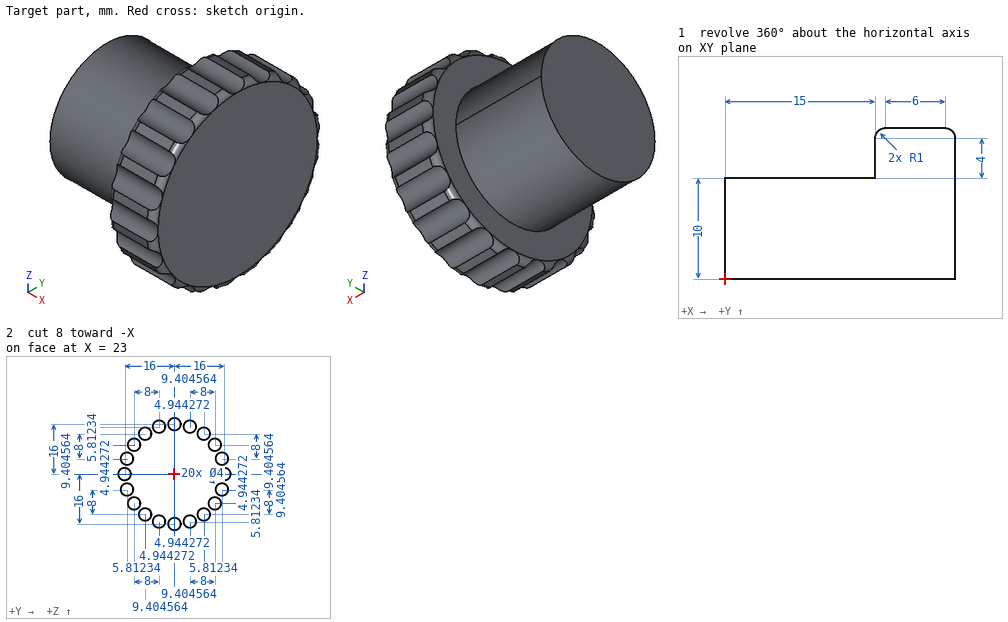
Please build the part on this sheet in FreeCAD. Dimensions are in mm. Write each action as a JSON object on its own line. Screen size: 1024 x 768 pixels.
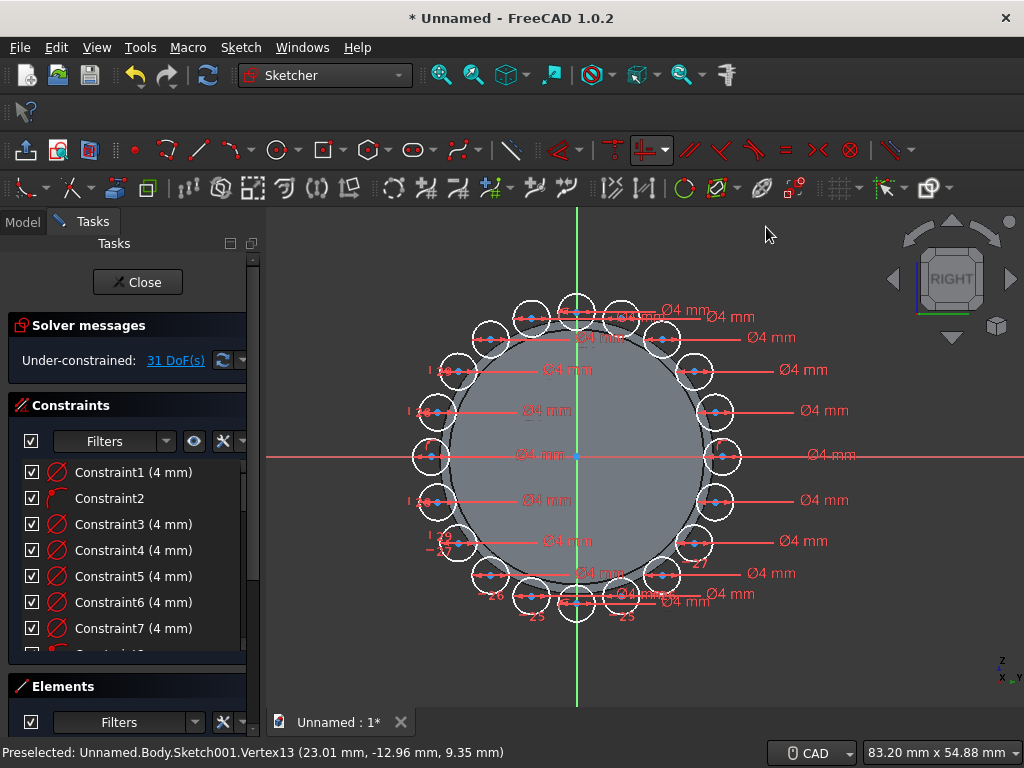
{"action": "left_click", "coordinate": [491, 575]}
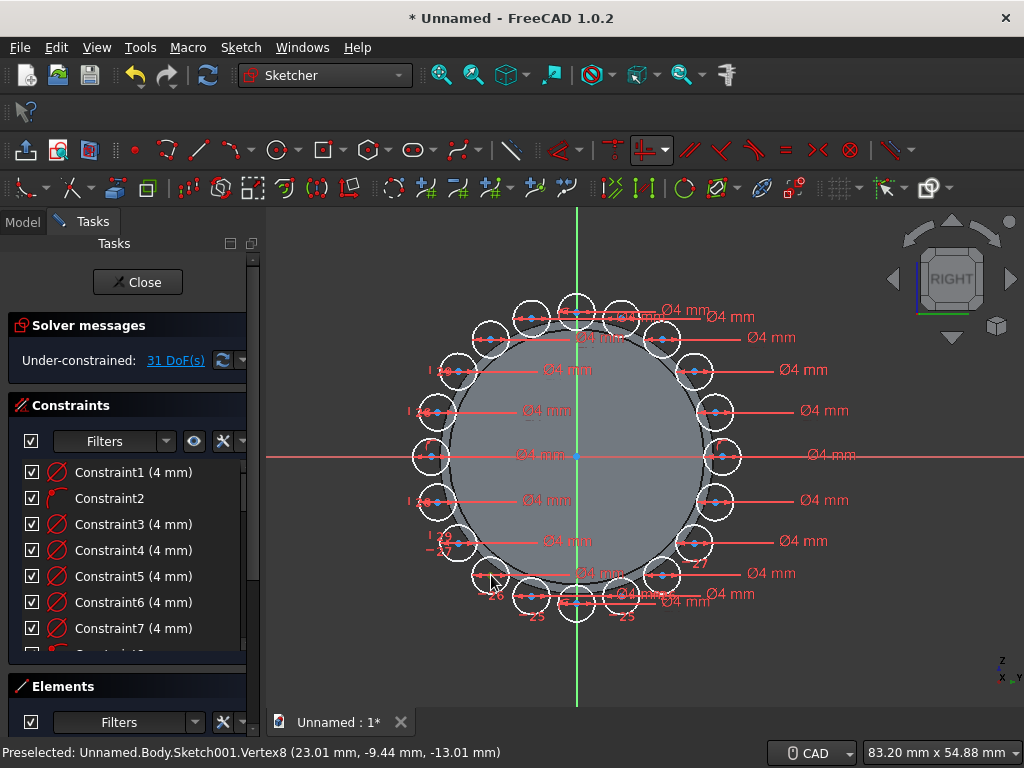
{"action": "left_click", "coordinate": [491, 340]}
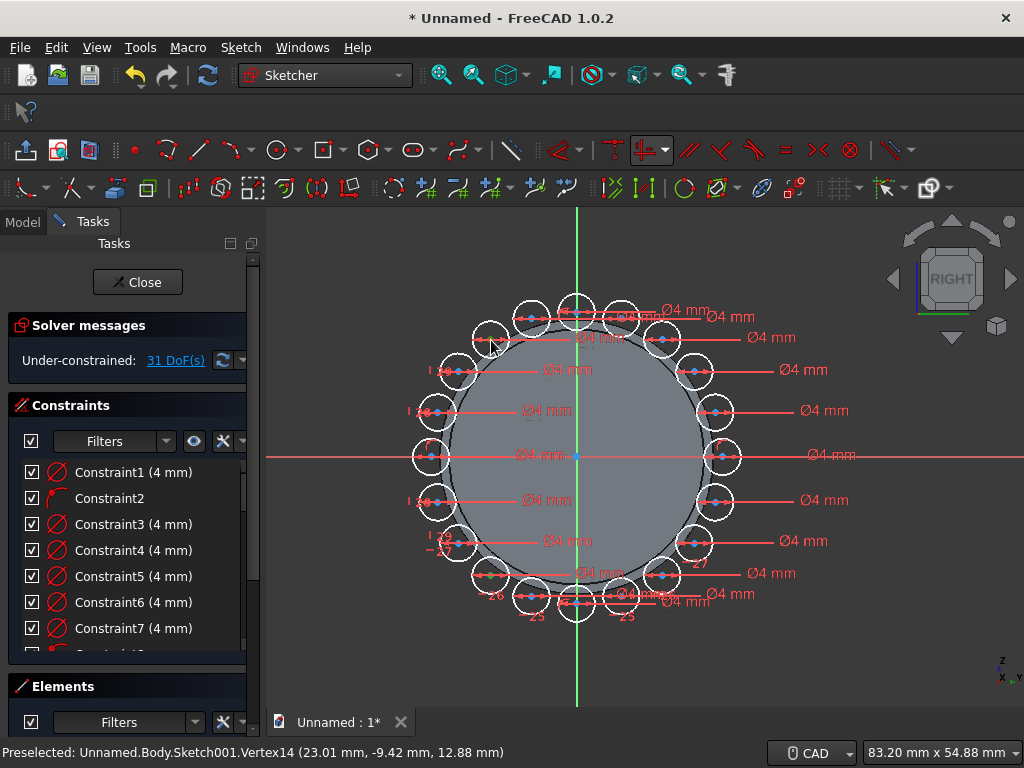
{"action": "left_click", "coordinate": [668, 150]}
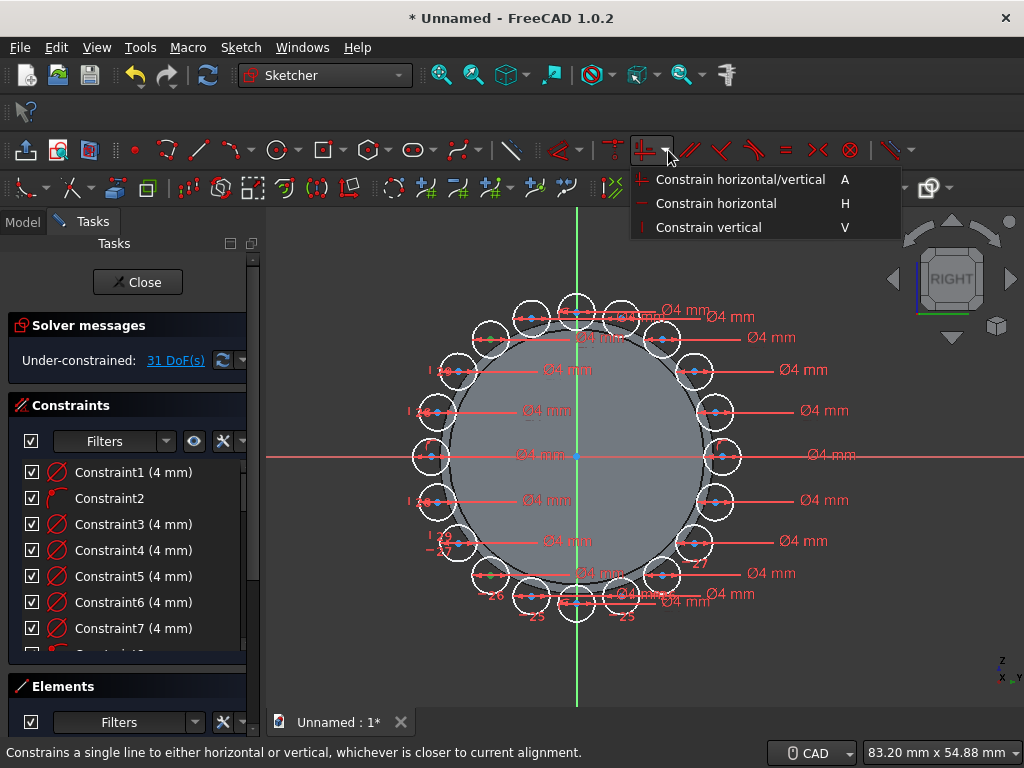
{"action": "left_click", "coordinate": [766, 227]}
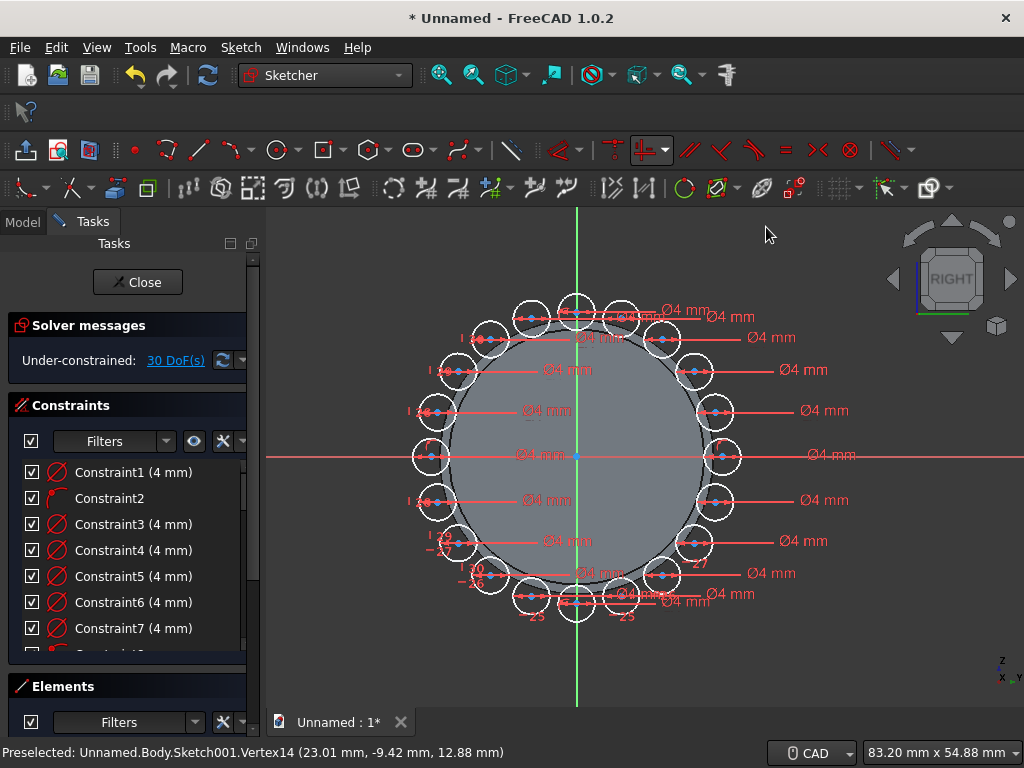
{"action": "left_click", "coordinate": [532, 319]}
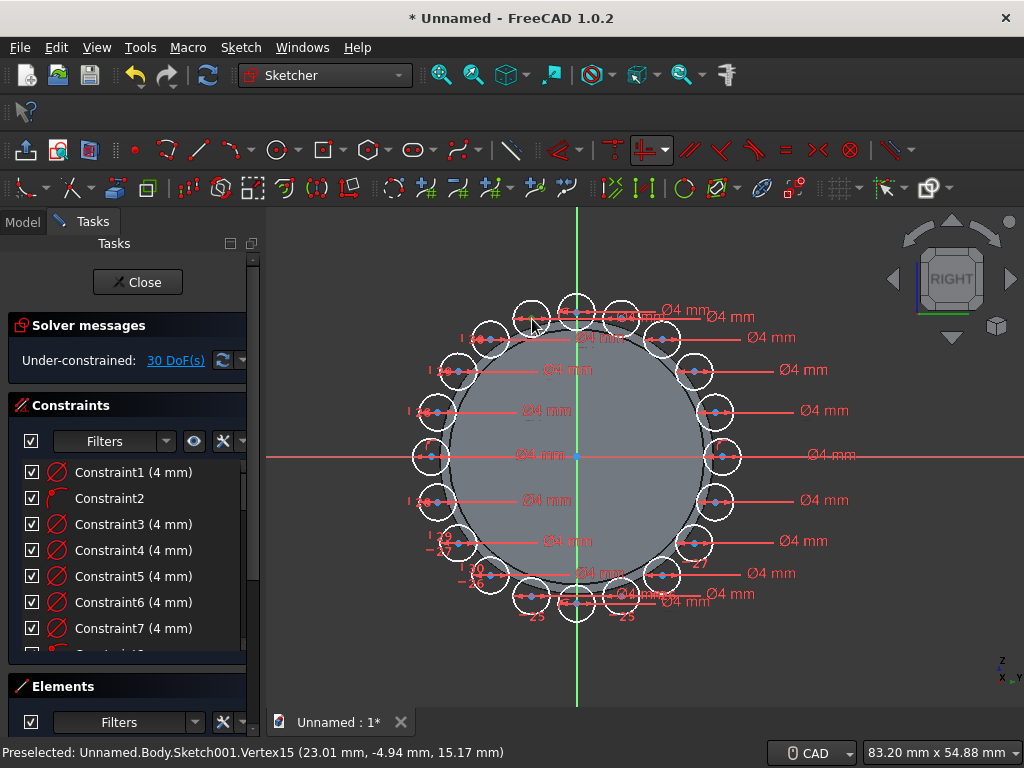
{"action": "left_click", "coordinate": [621, 319]}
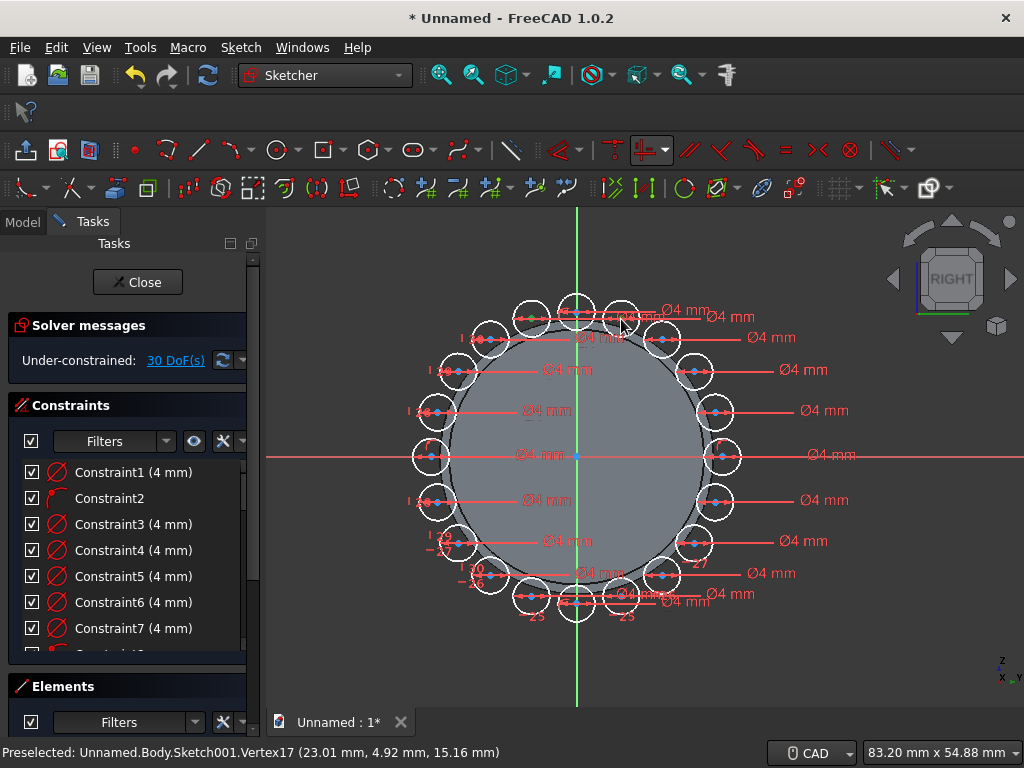
{"action": "left_click", "coordinate": [668, 150]}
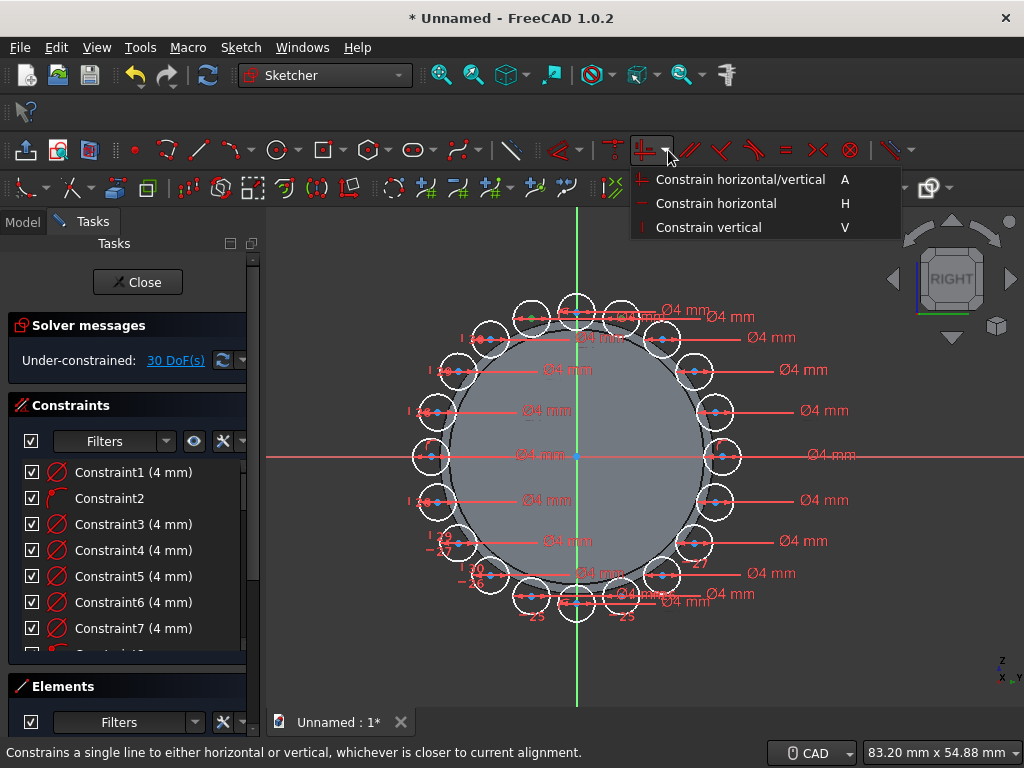
{"action": "left_click", "coordinate": [766, 203]}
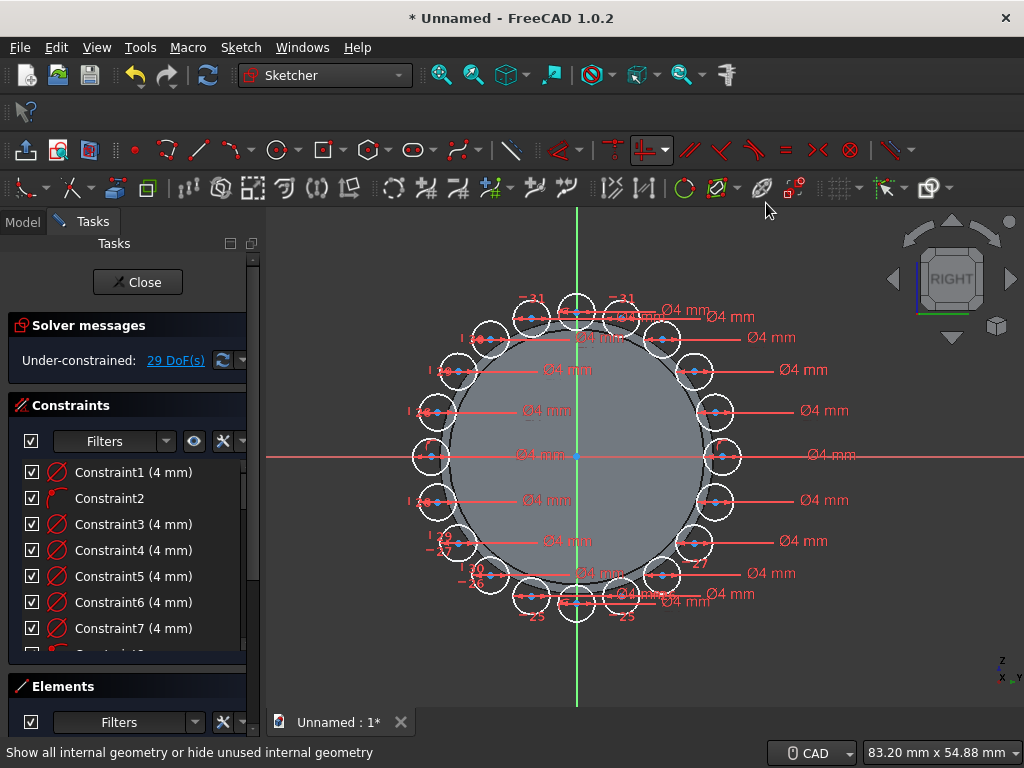
{"action": "left_click", "coordinate": [491, 340]}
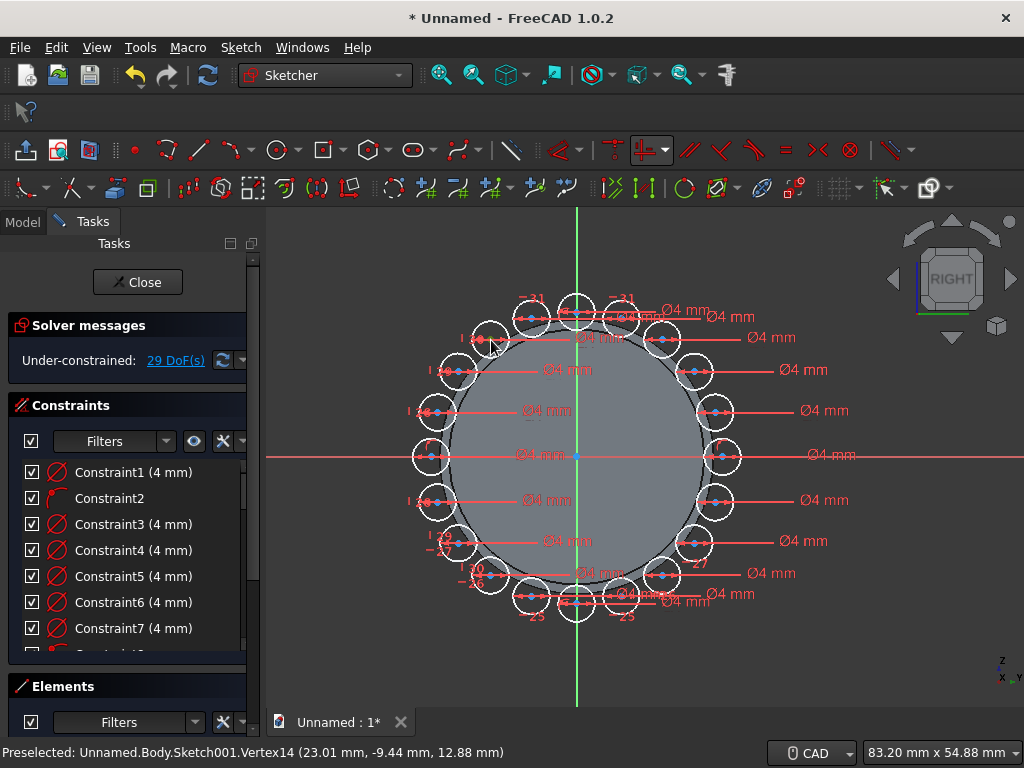
{"action": "left_click", "coordinate": [662, 340]}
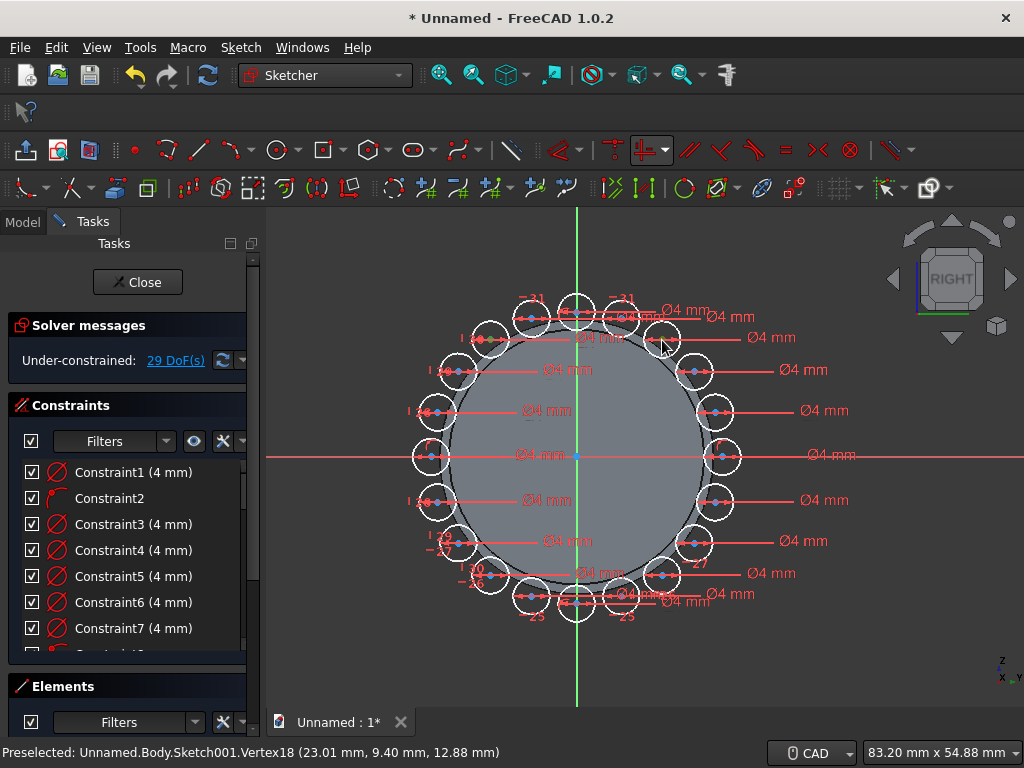
{"action": "key", "text": "h"}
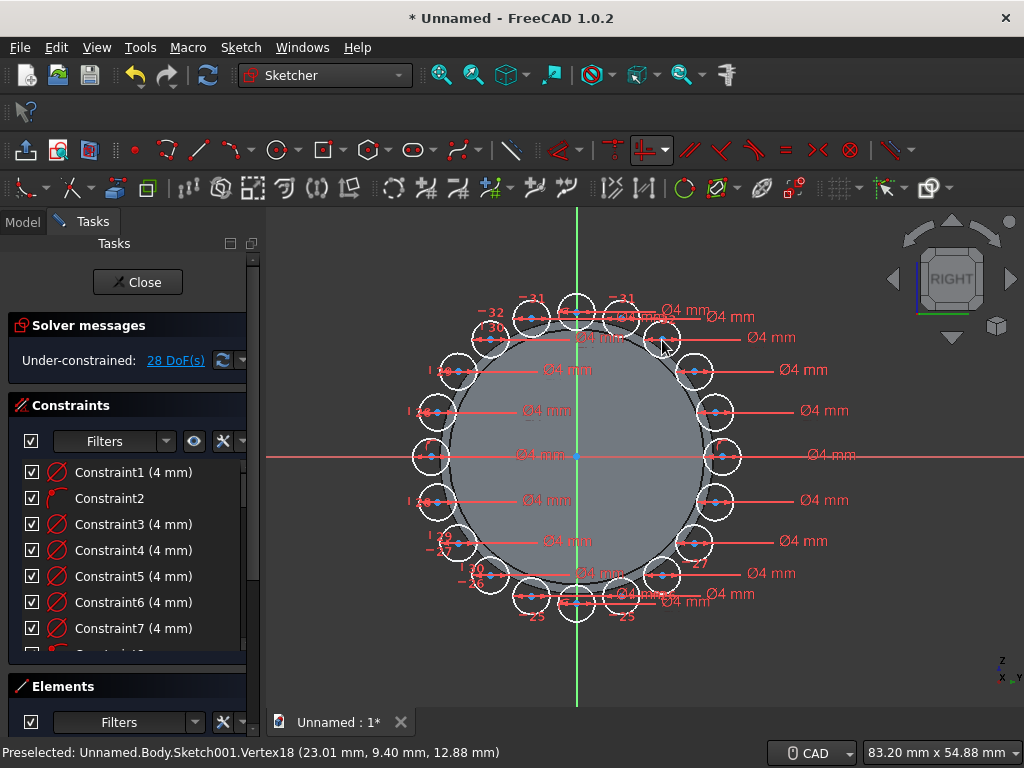
{"action": "left_click", "coordinate": [715, 502]}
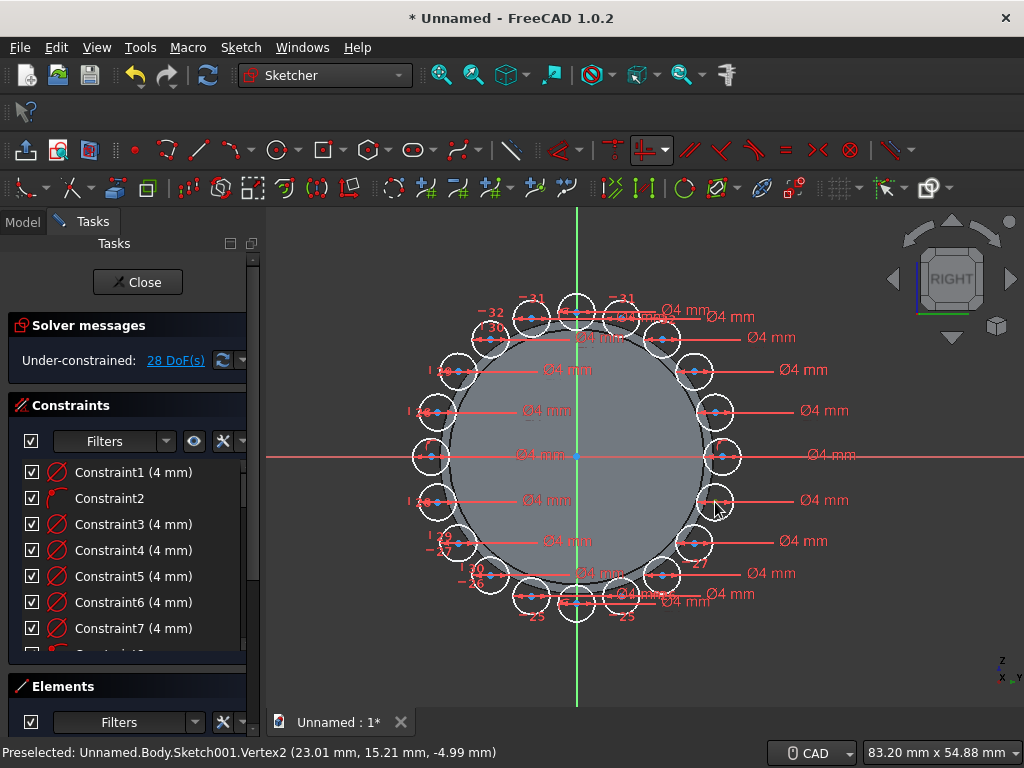
{"action": "left_click", "coordinate": [715, 413]}